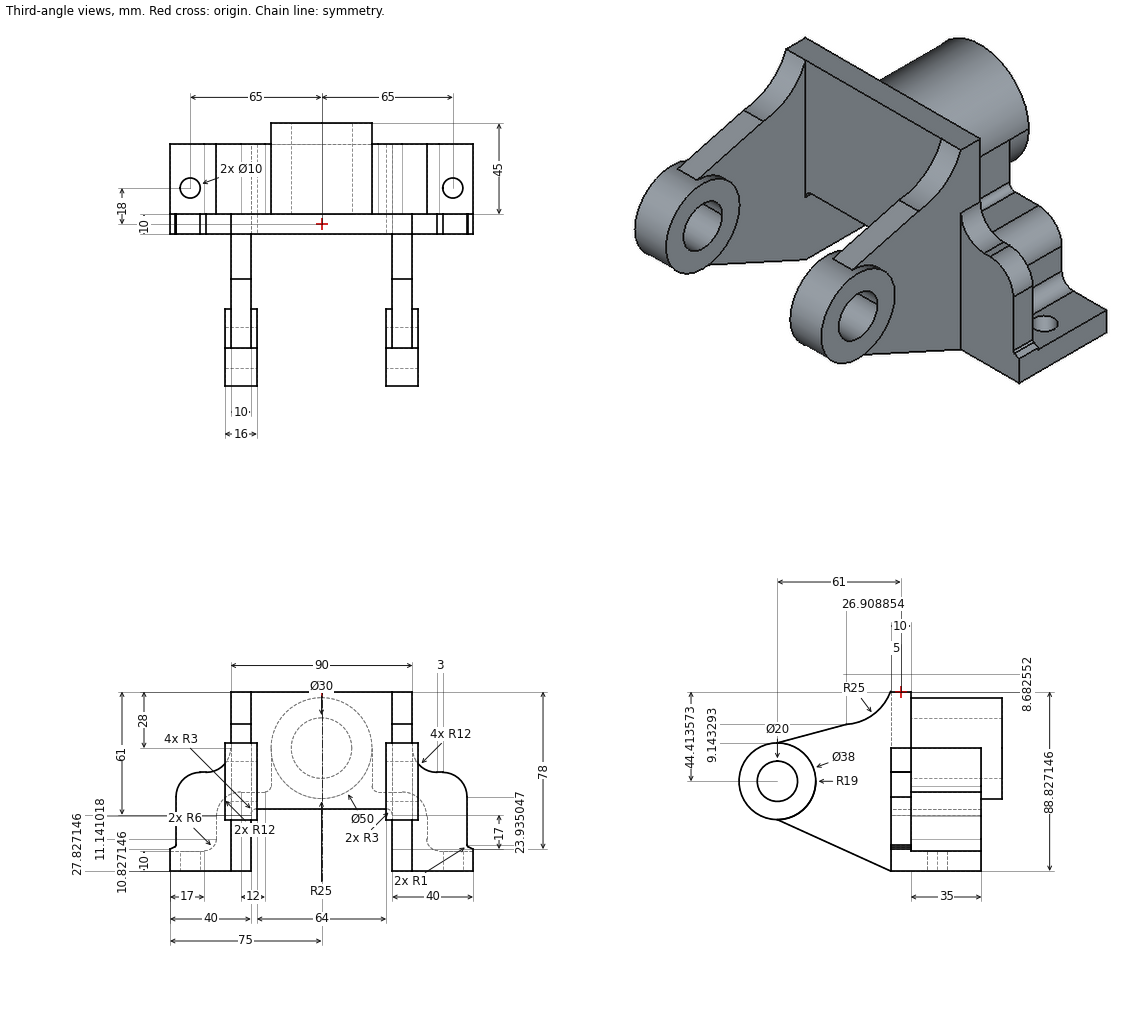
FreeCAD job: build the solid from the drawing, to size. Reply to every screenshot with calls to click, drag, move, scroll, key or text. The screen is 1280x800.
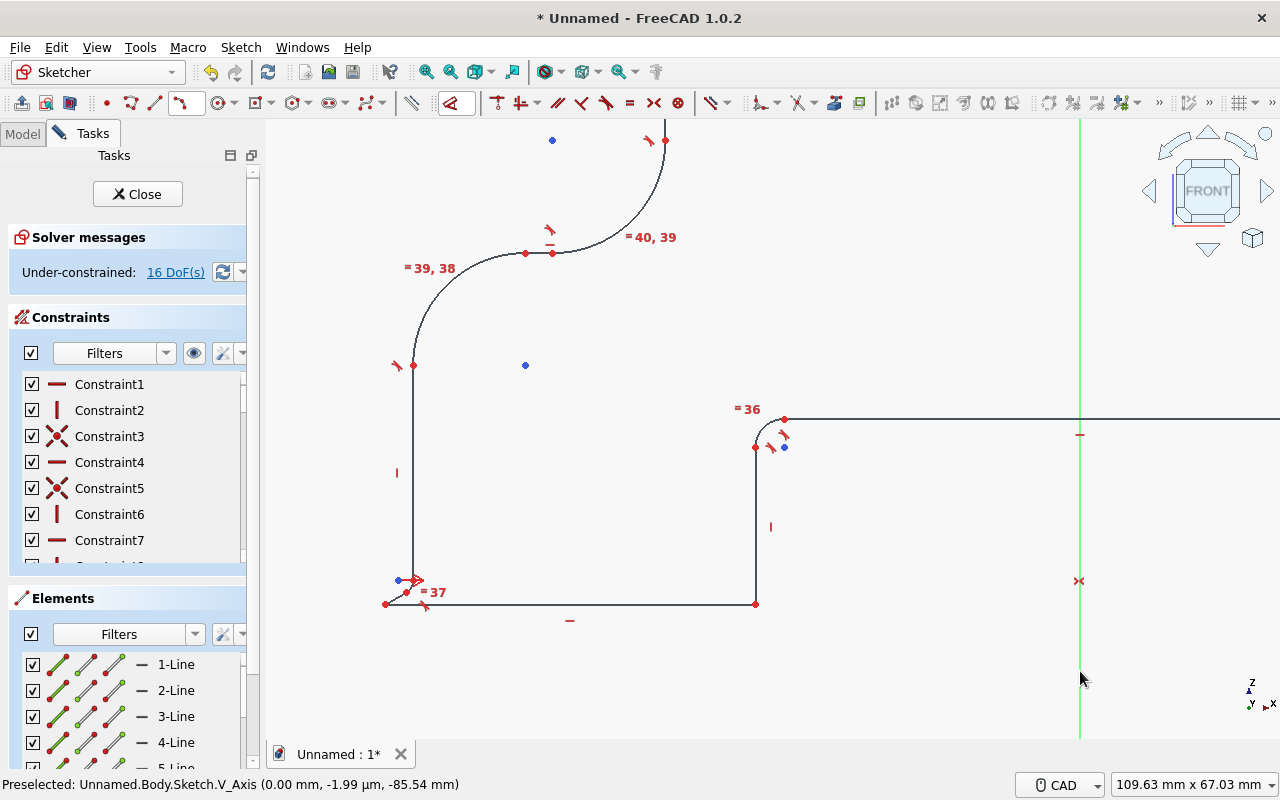
scroll(398, 582, down, 4)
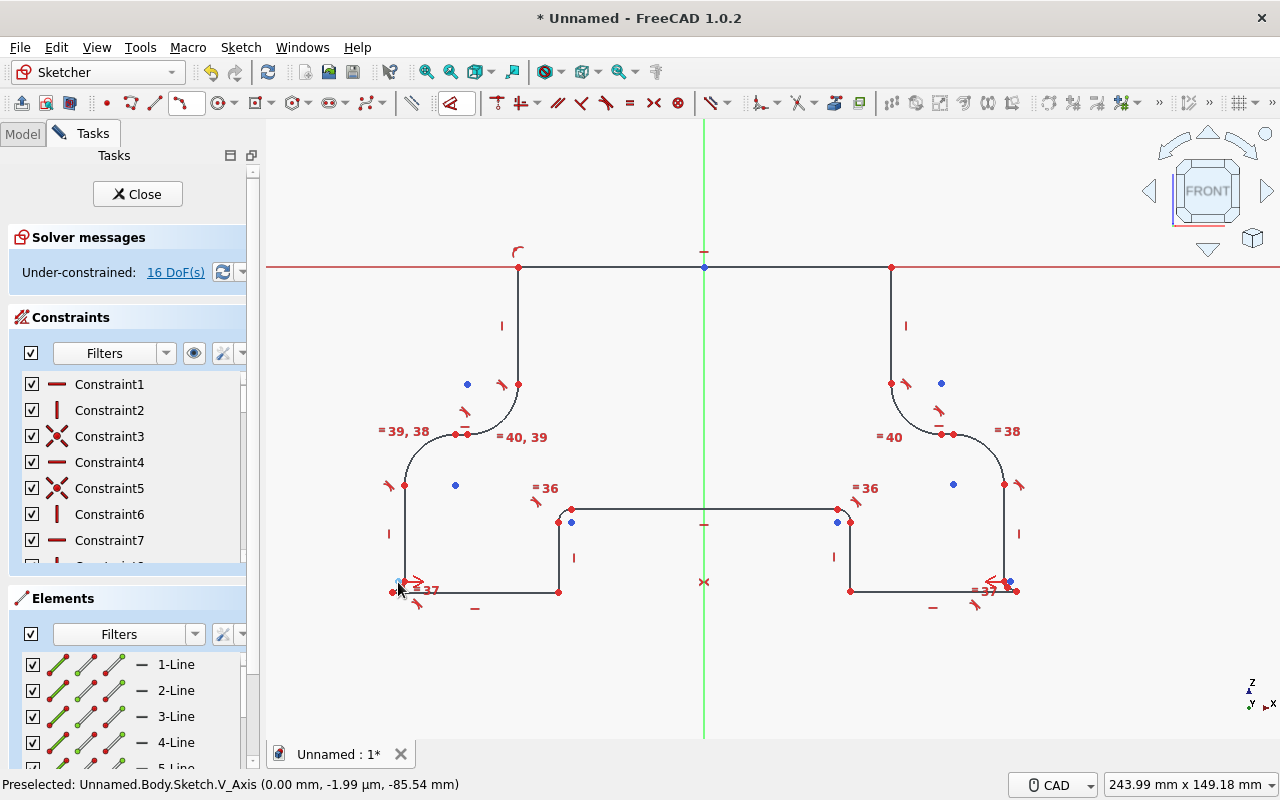
click(468, 384)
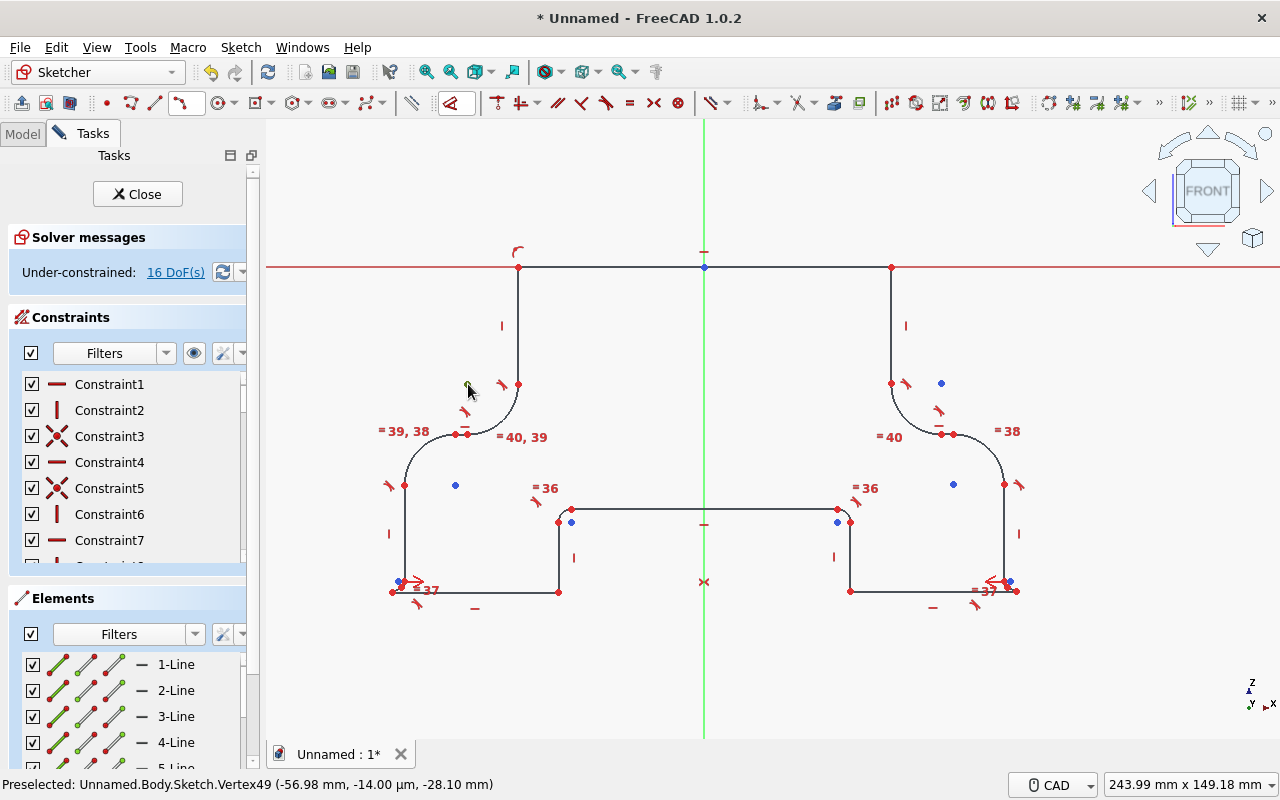
click(942, 384)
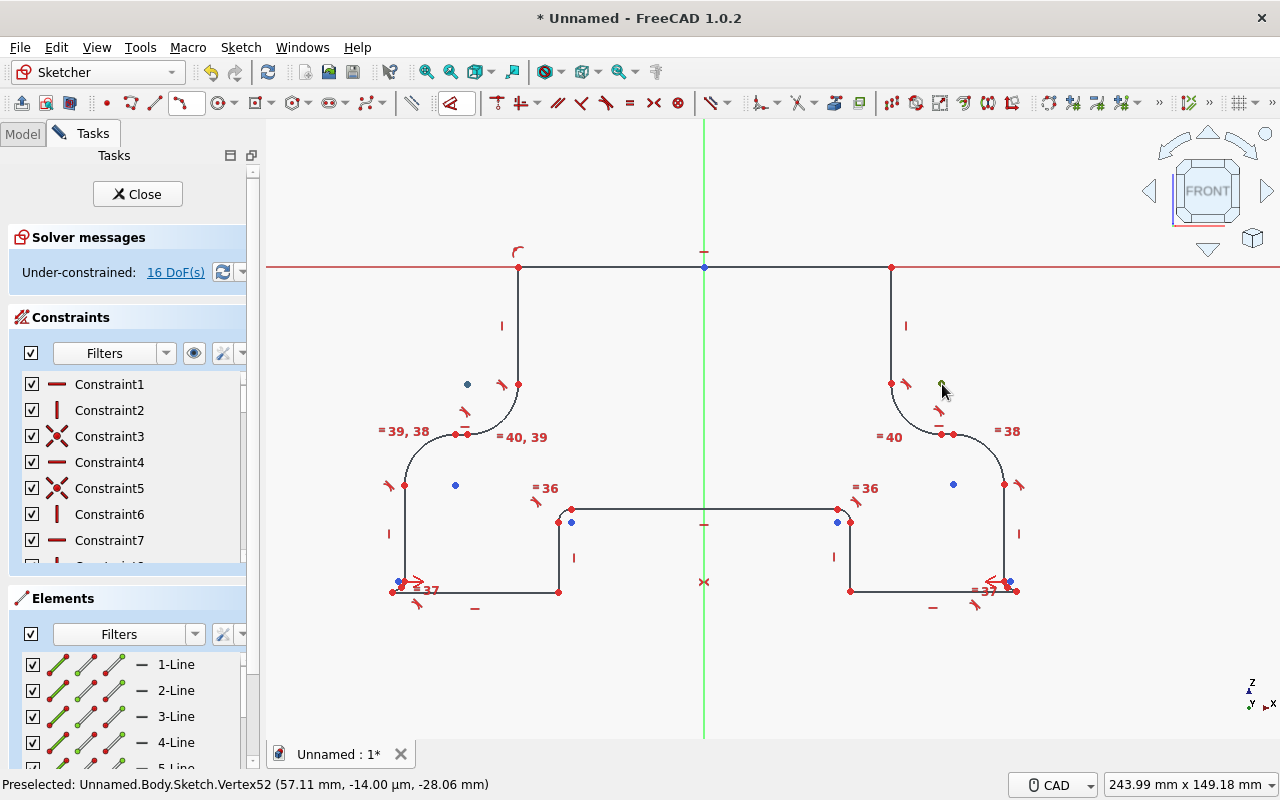
click(704, 671)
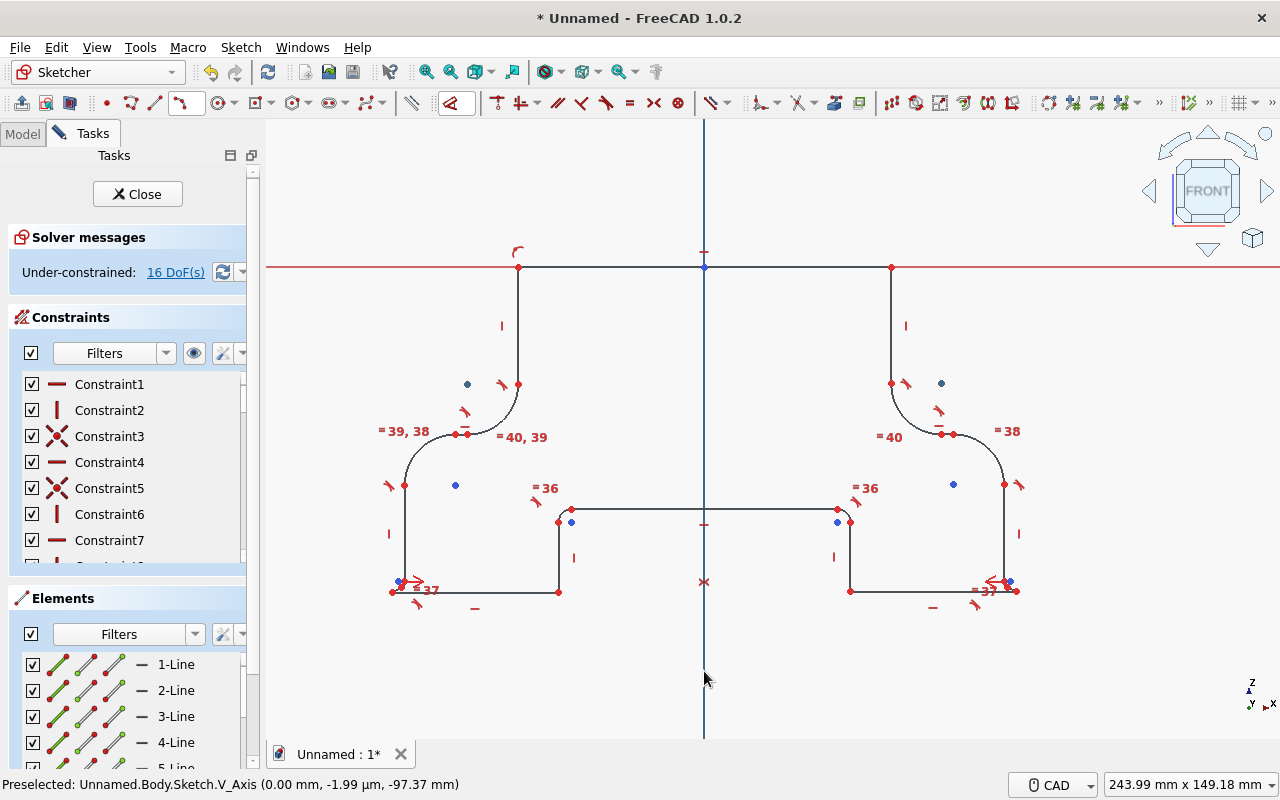
click(654, 104)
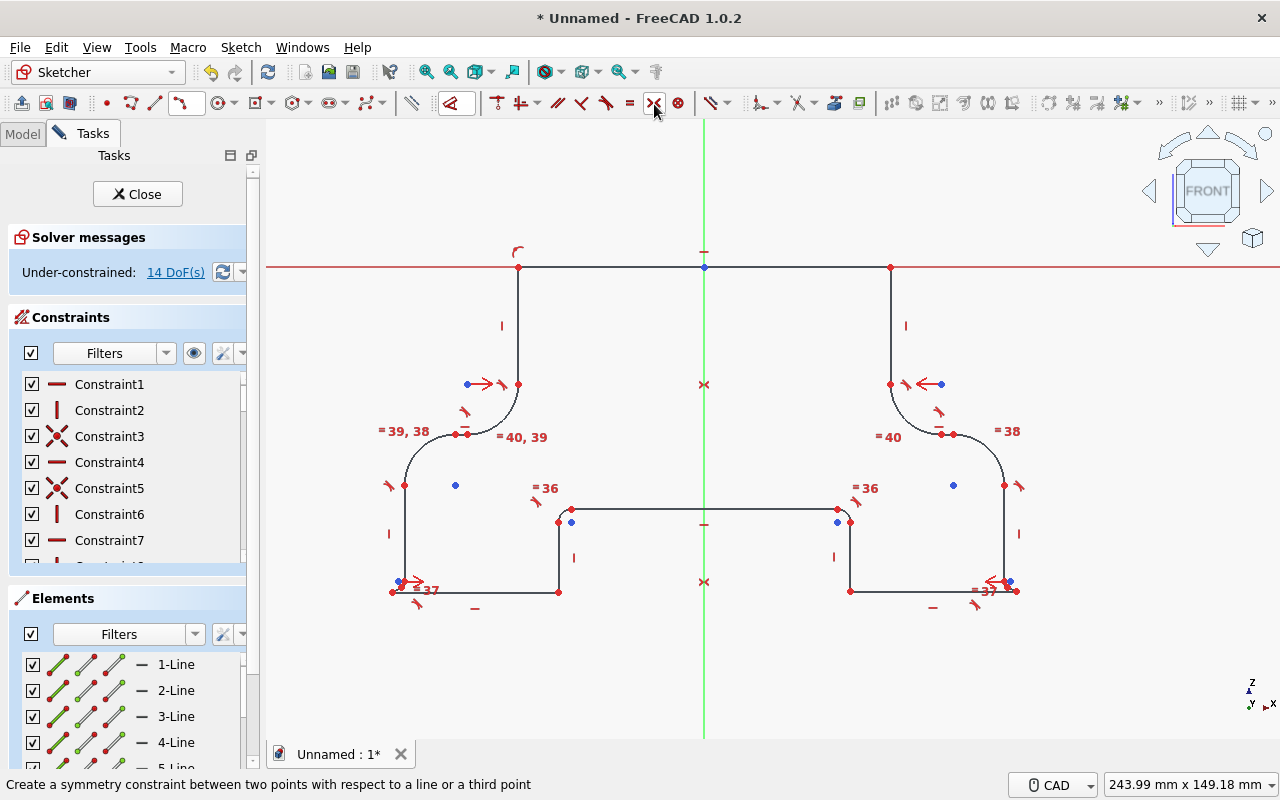
click(850, 592)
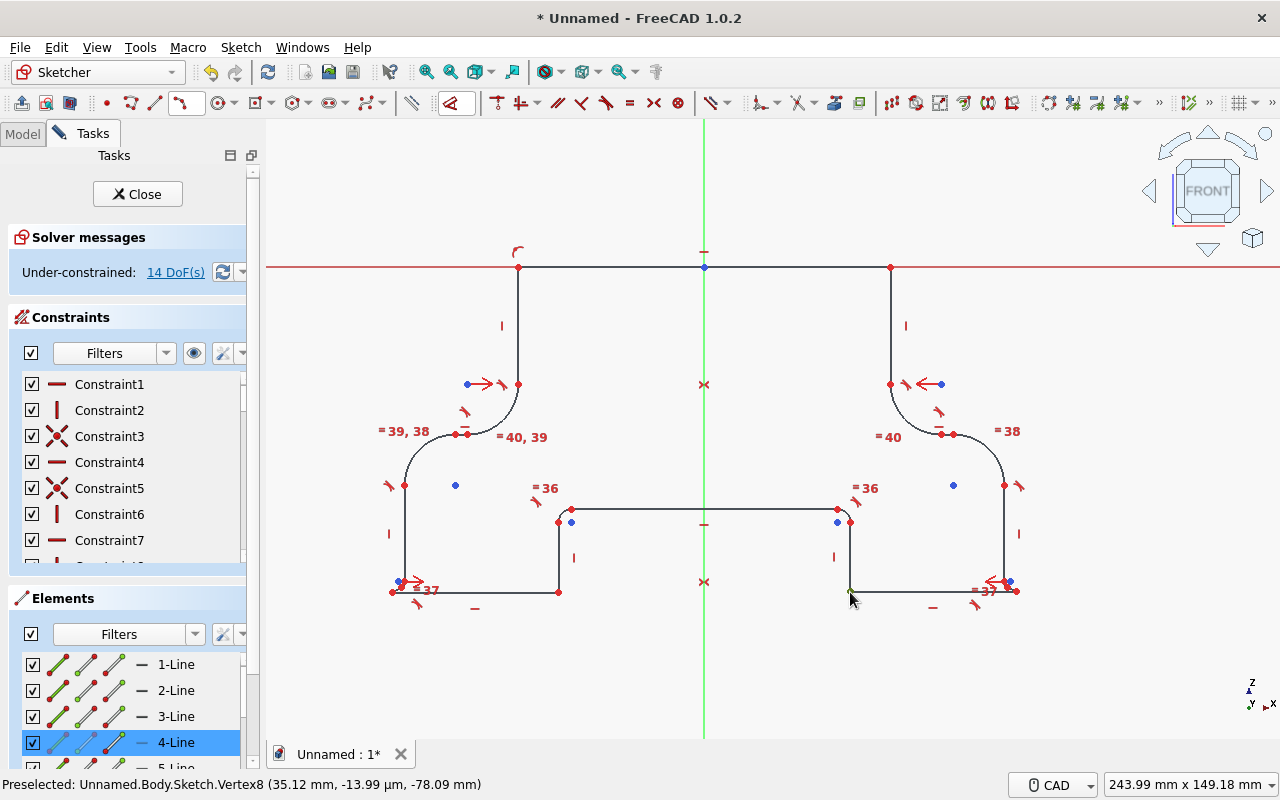
click(559, 593)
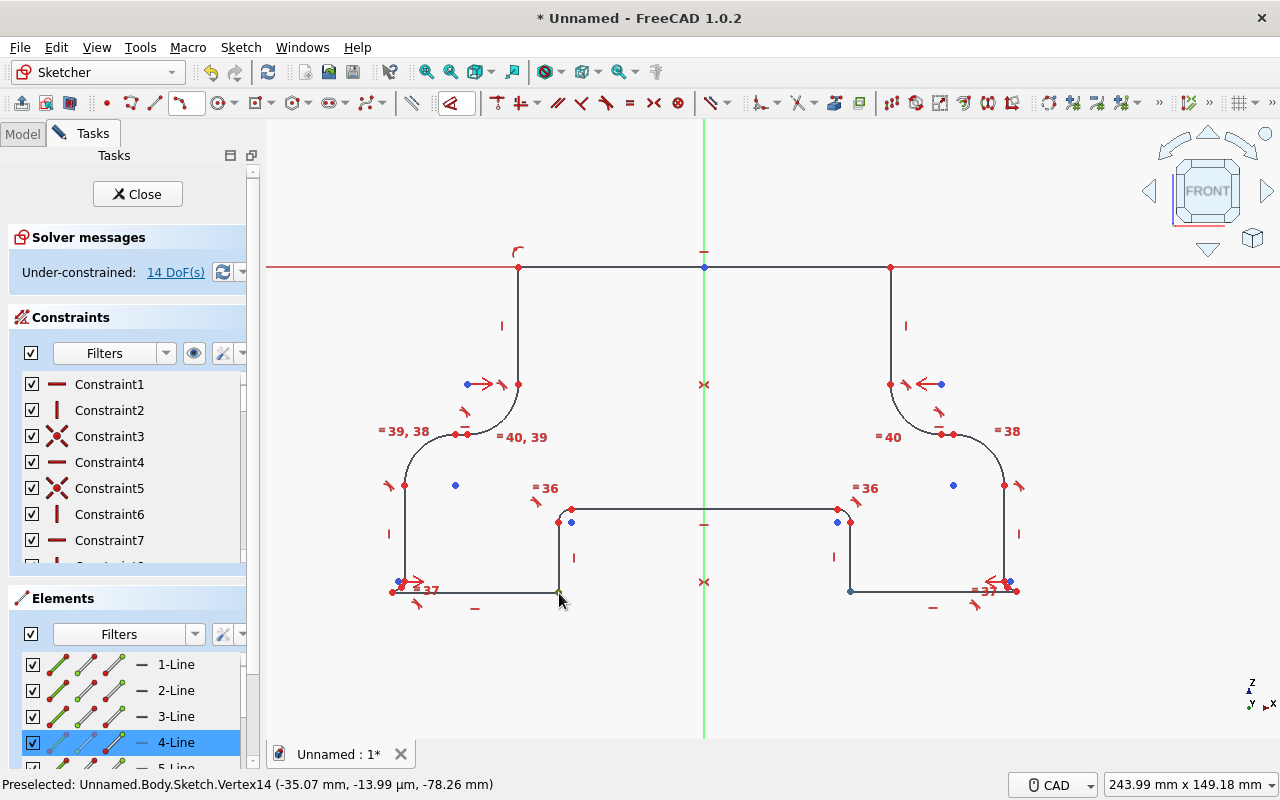
click(704, 671)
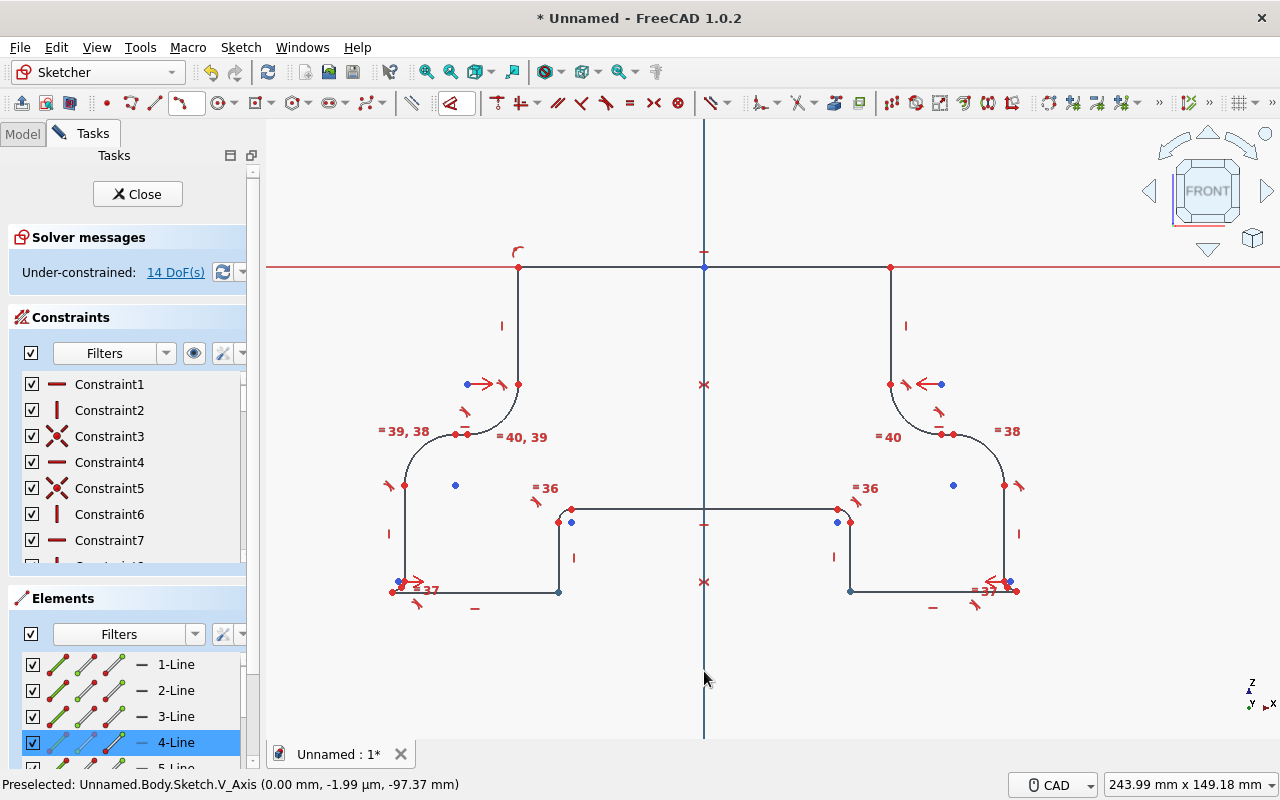
click(654, 104)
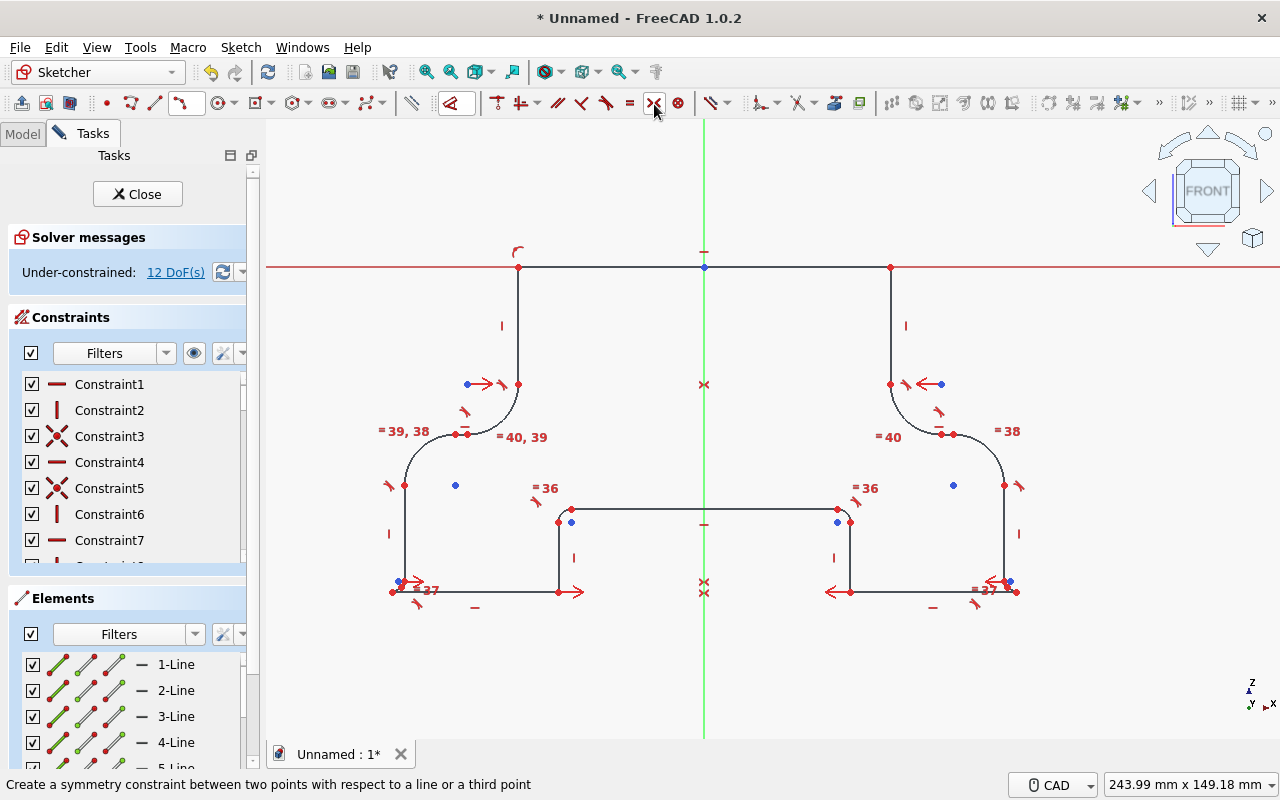
key(d)